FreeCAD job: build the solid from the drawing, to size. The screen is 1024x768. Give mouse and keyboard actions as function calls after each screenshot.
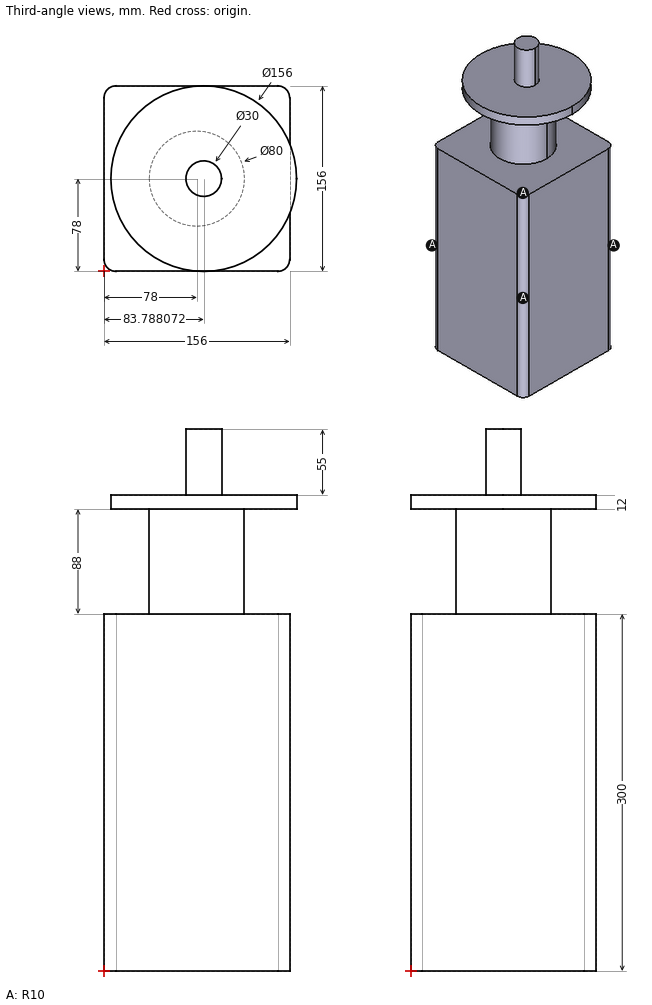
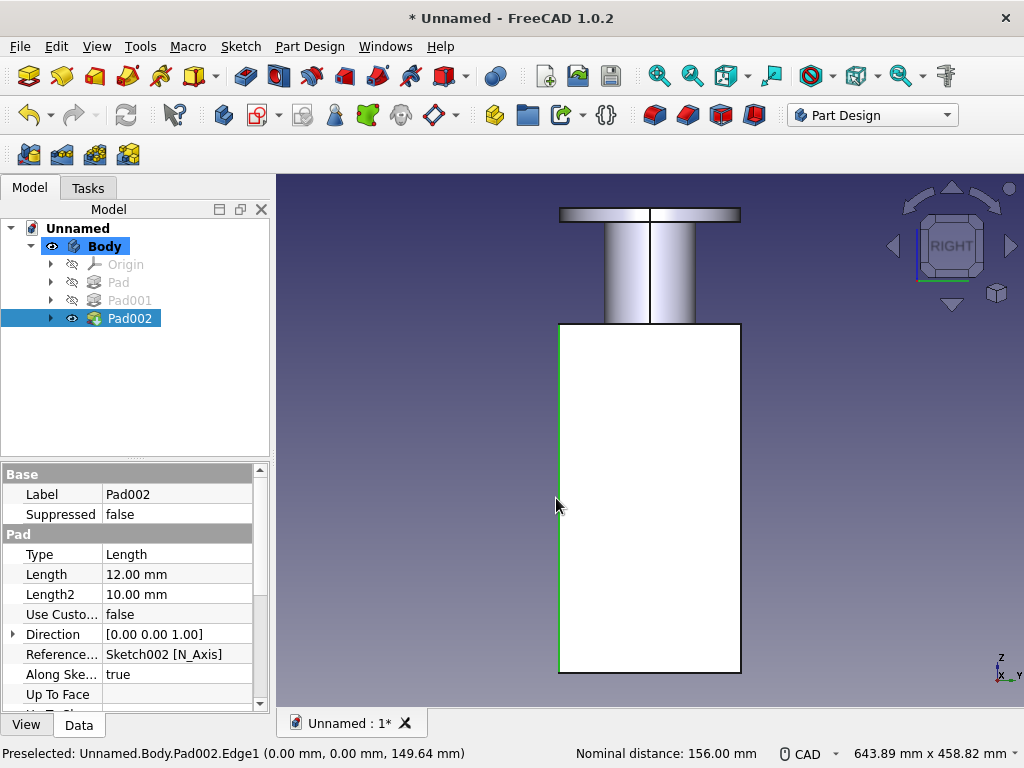
click(741, 498, ctrl)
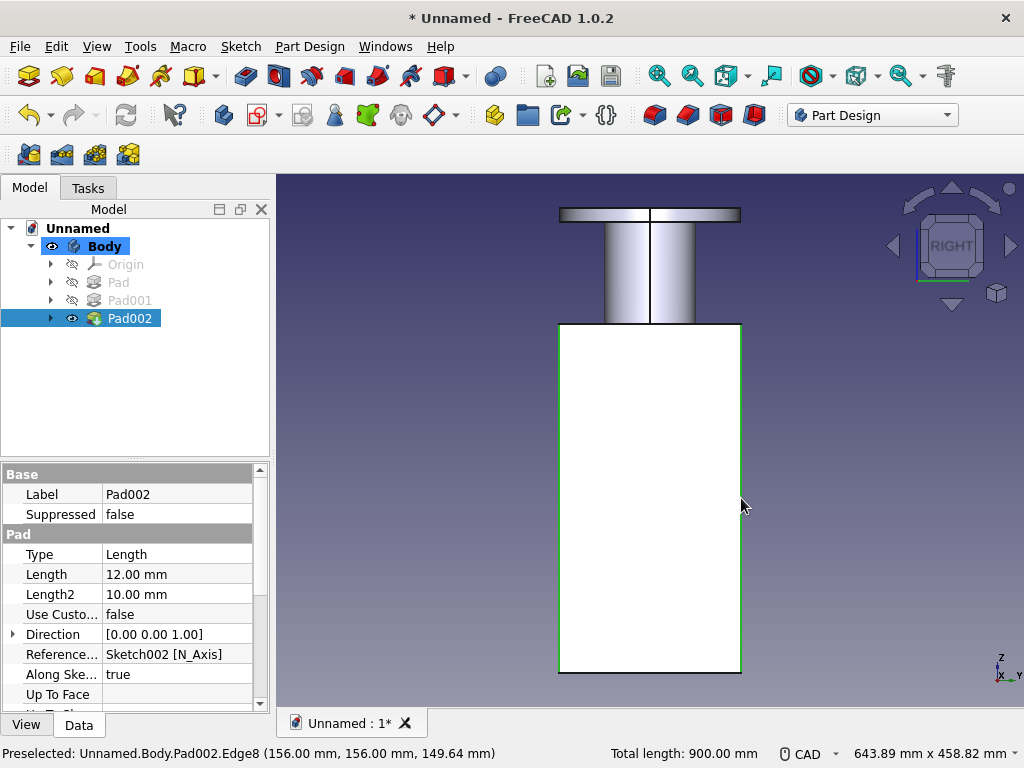
key(5)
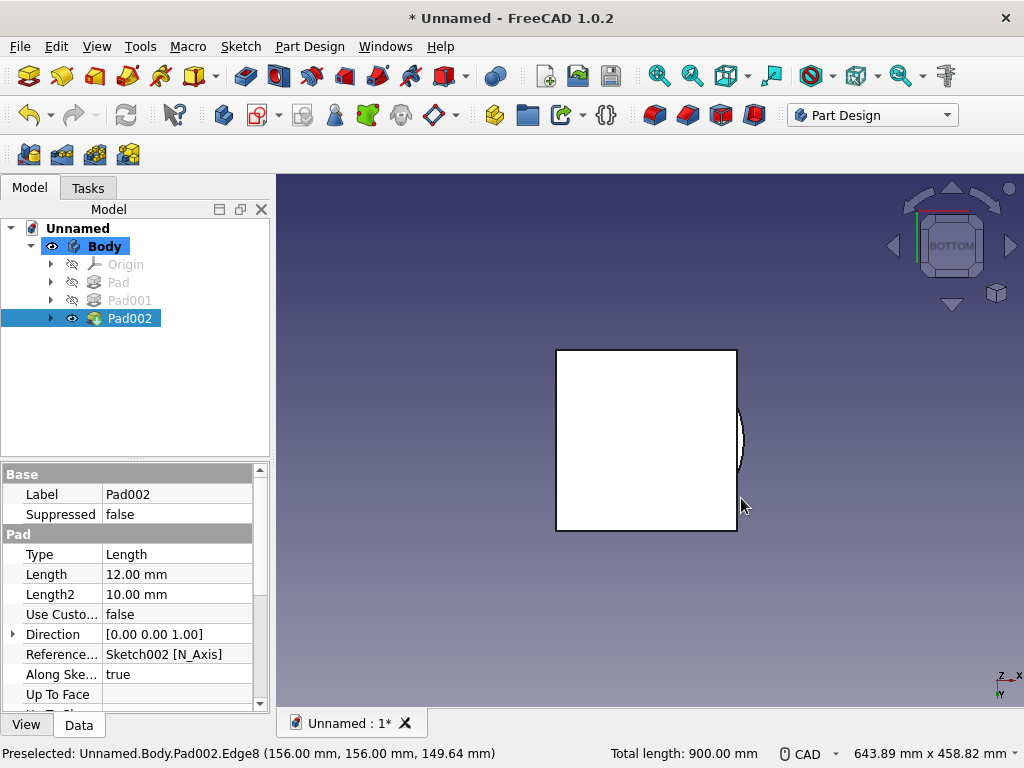
click(660, 76)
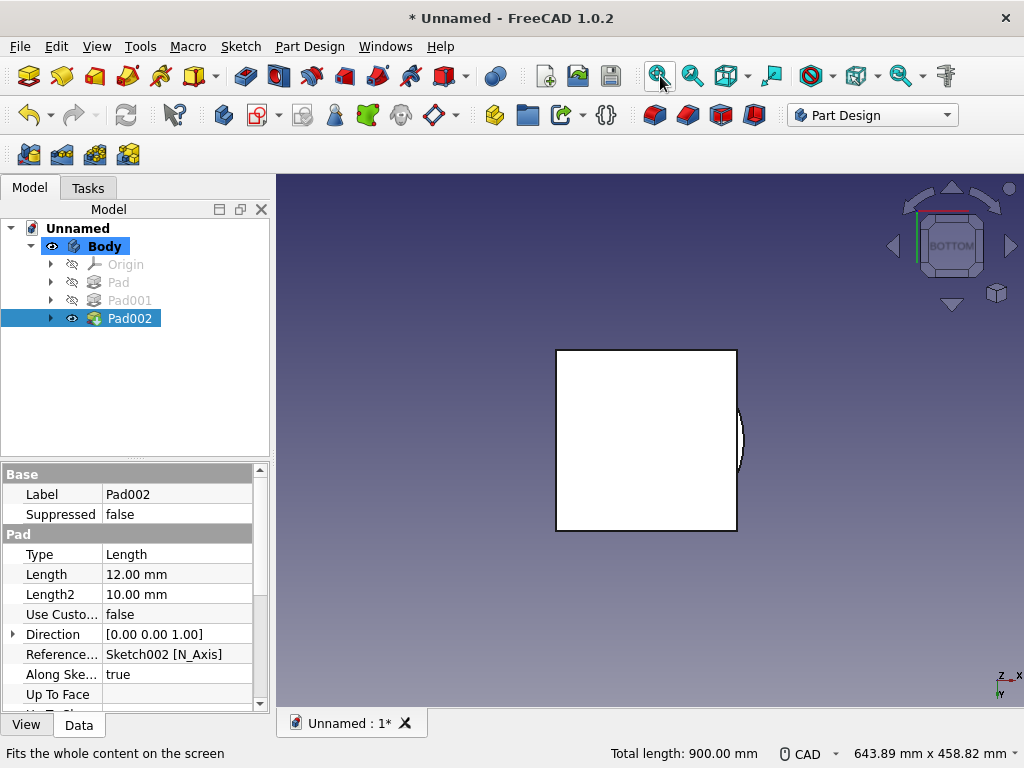
key(4)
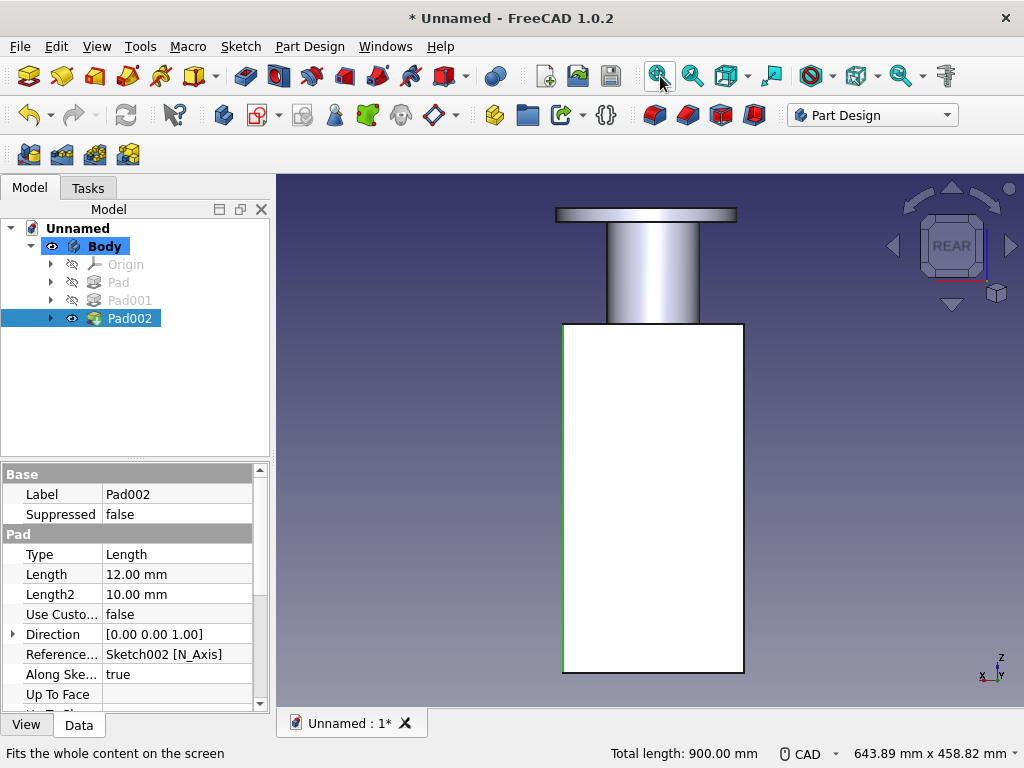
click(744, 498, ctrl)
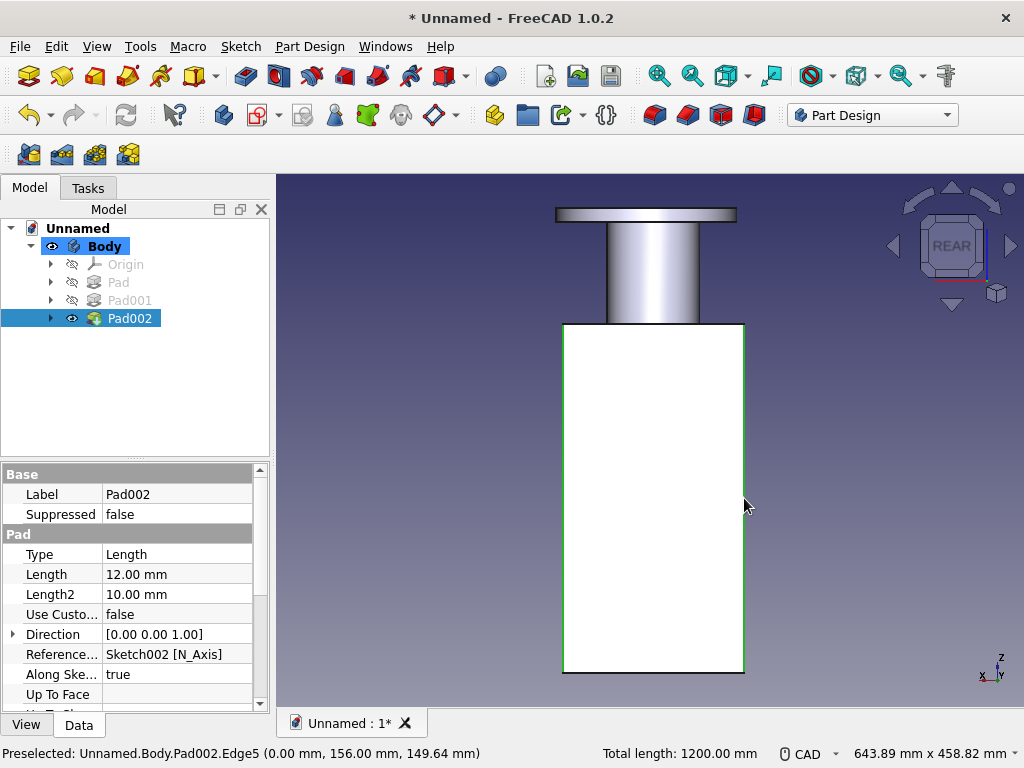
click(655, 116)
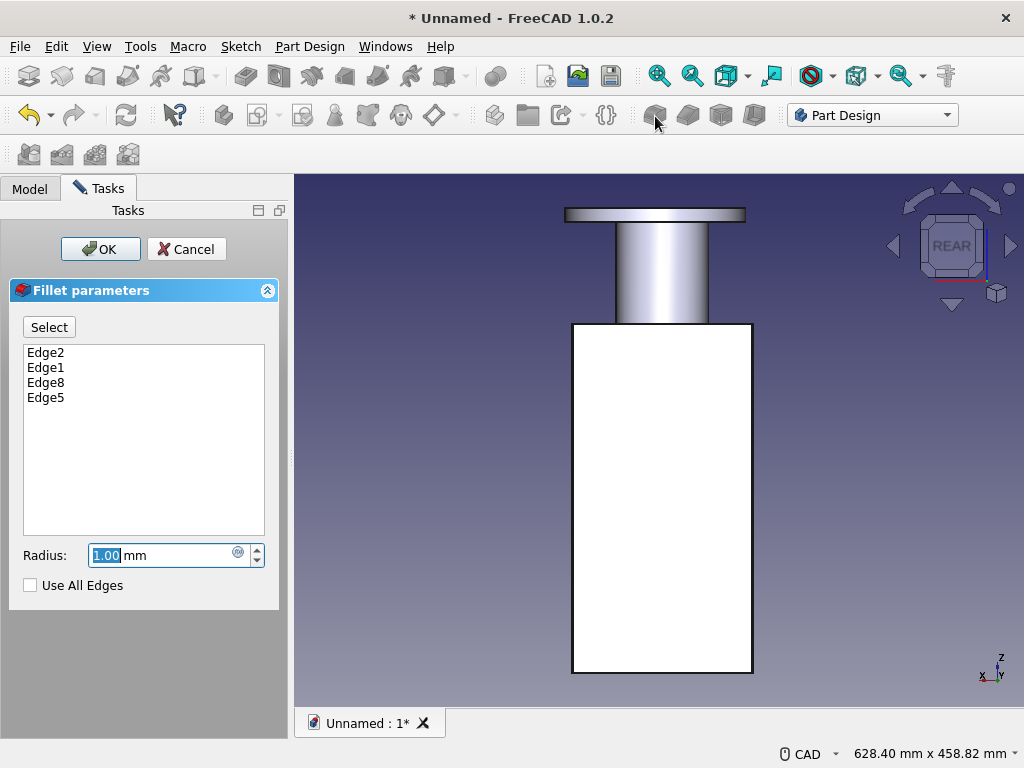
text(10)
key(Tab)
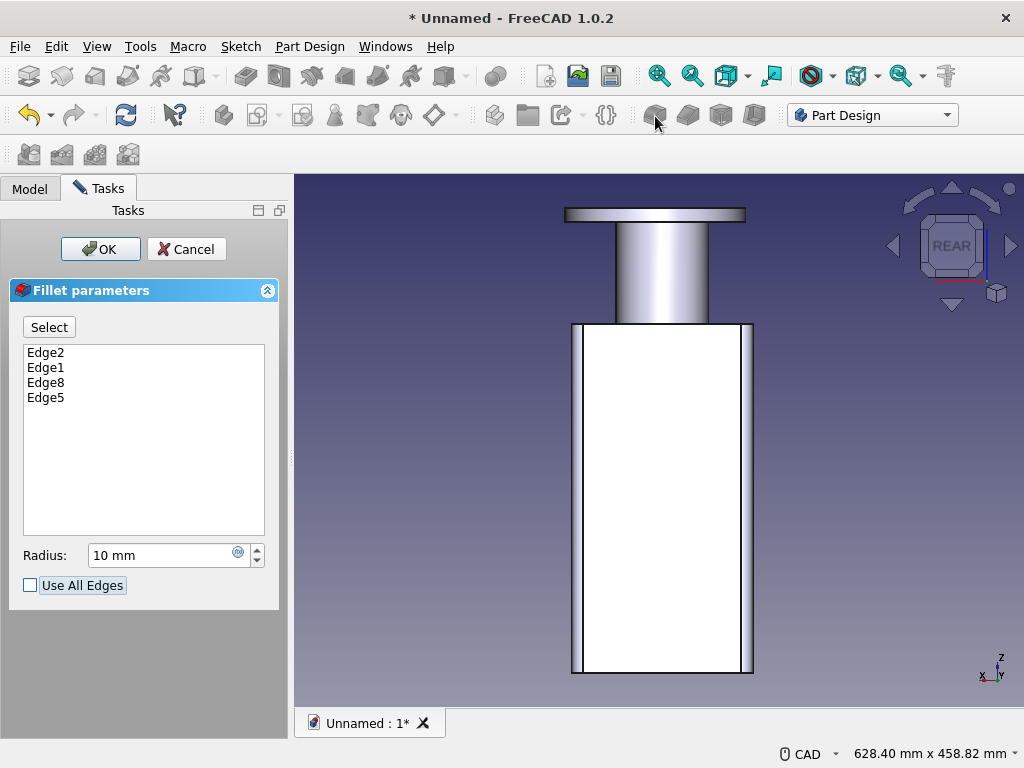
click(101, 249)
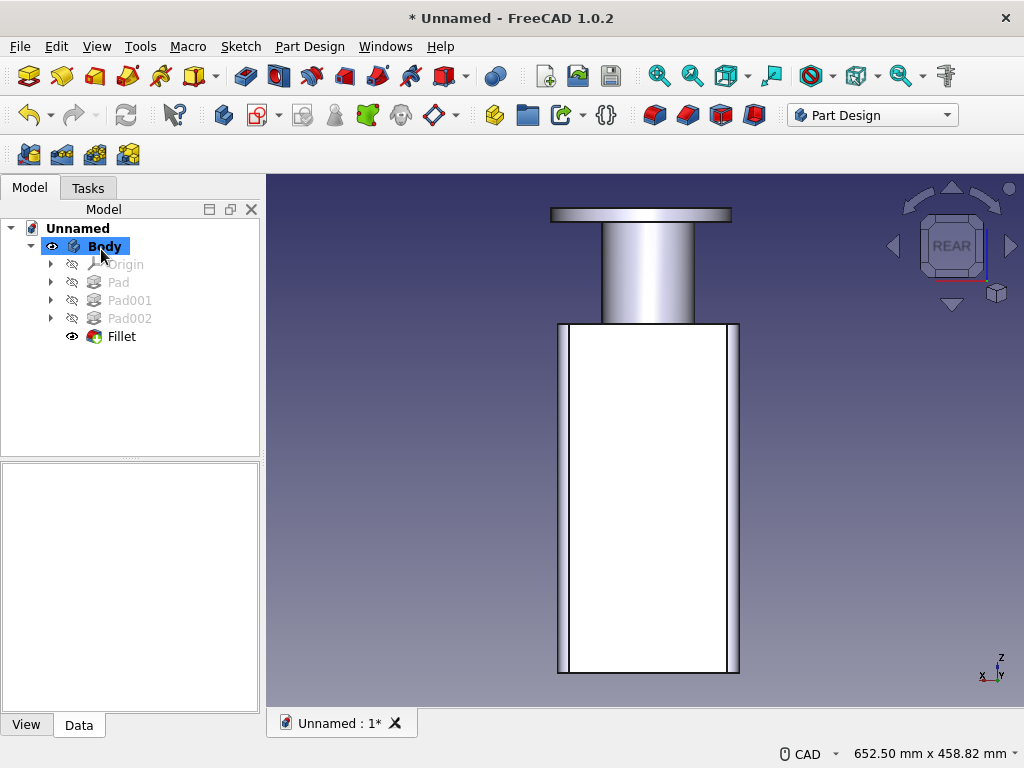
key(0)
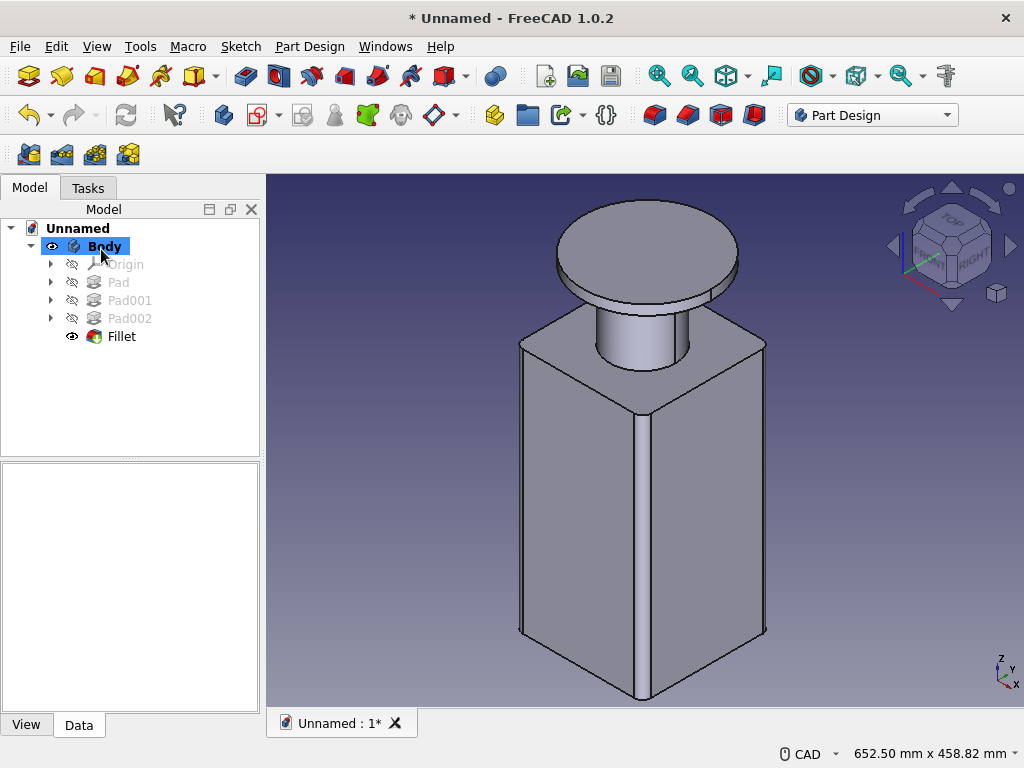
click(647, 251)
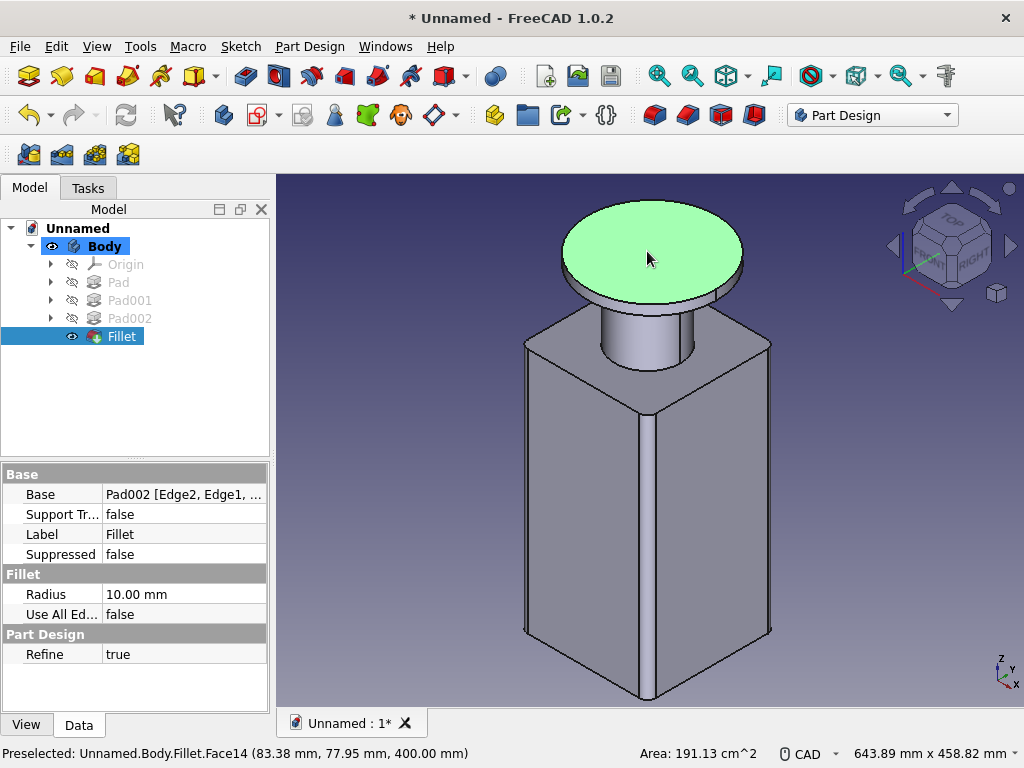
click(256, 116)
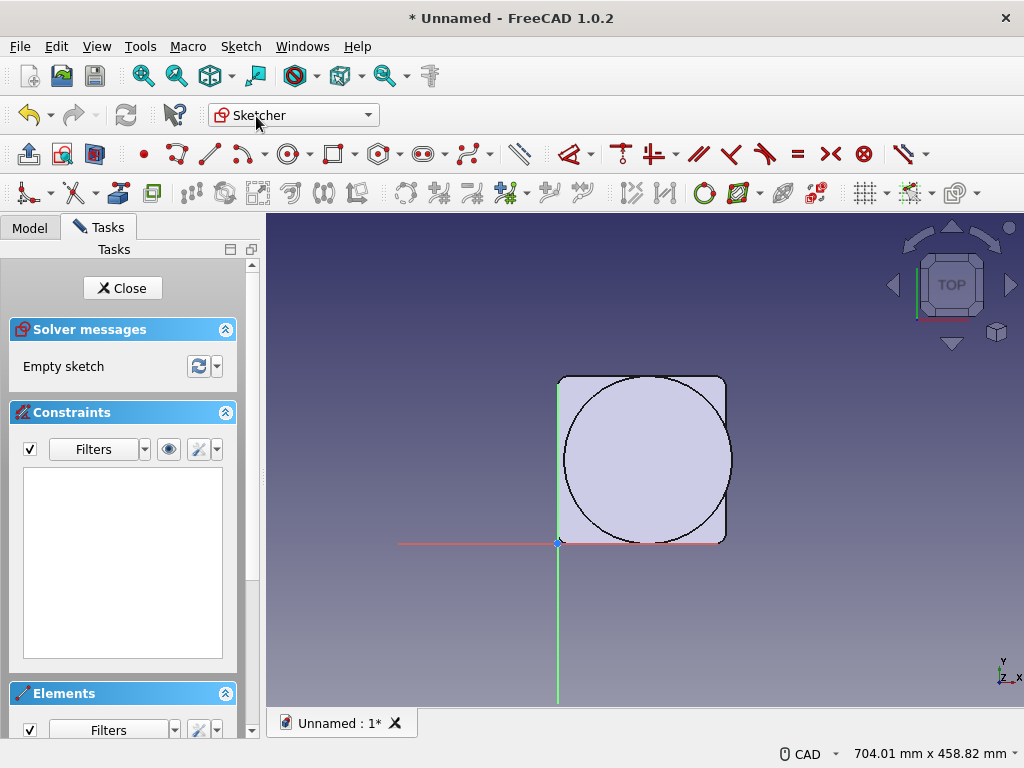
scroll(657, 460, up, 11)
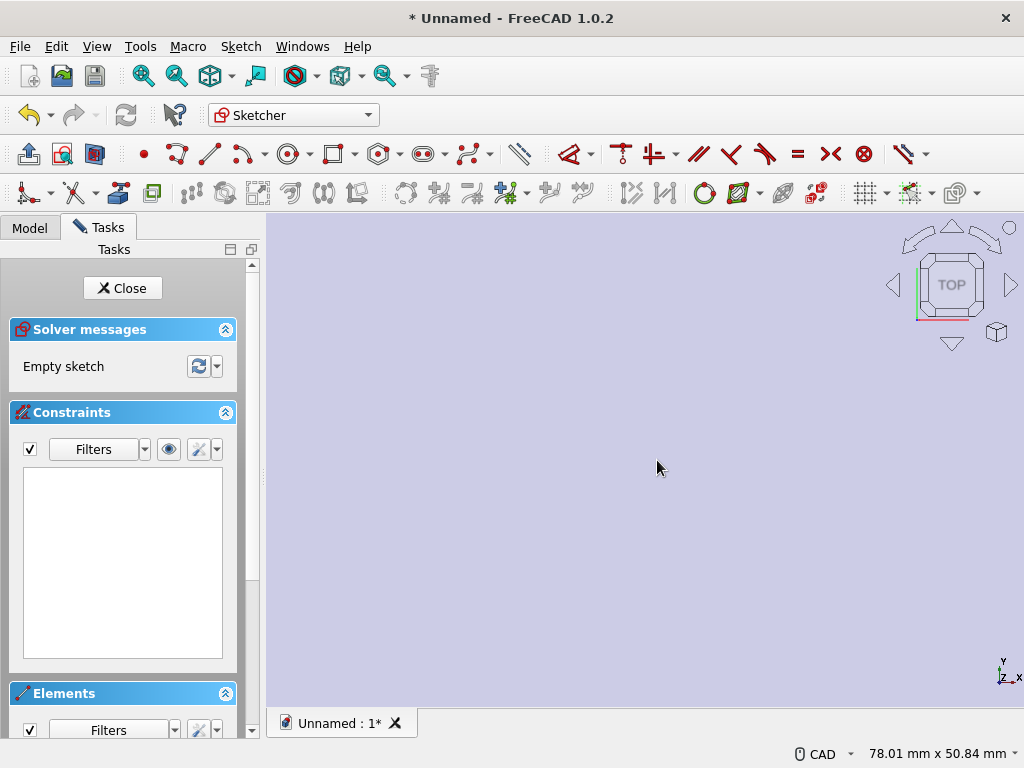
click(288, 154)